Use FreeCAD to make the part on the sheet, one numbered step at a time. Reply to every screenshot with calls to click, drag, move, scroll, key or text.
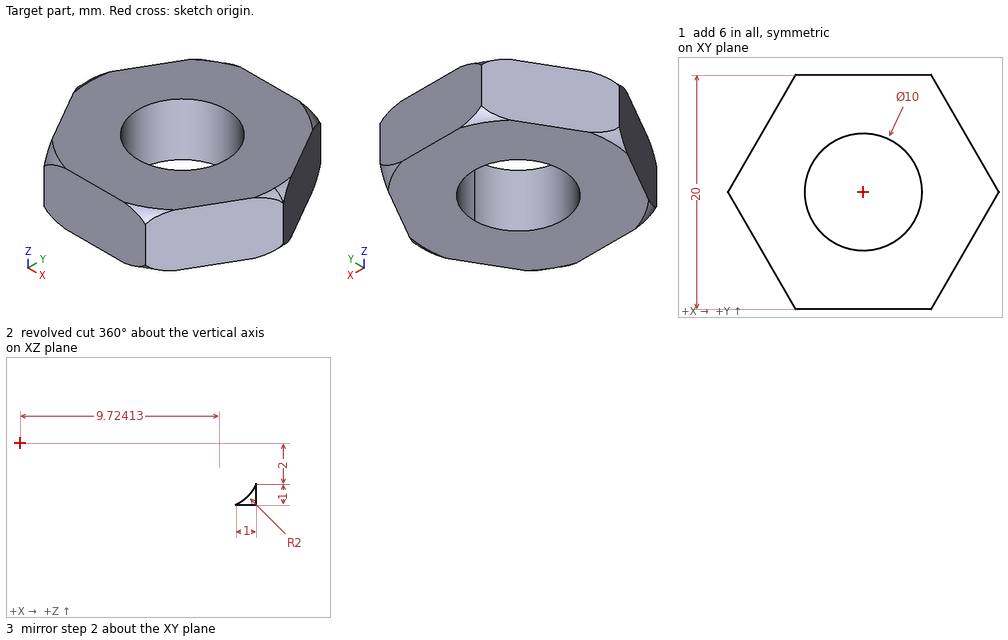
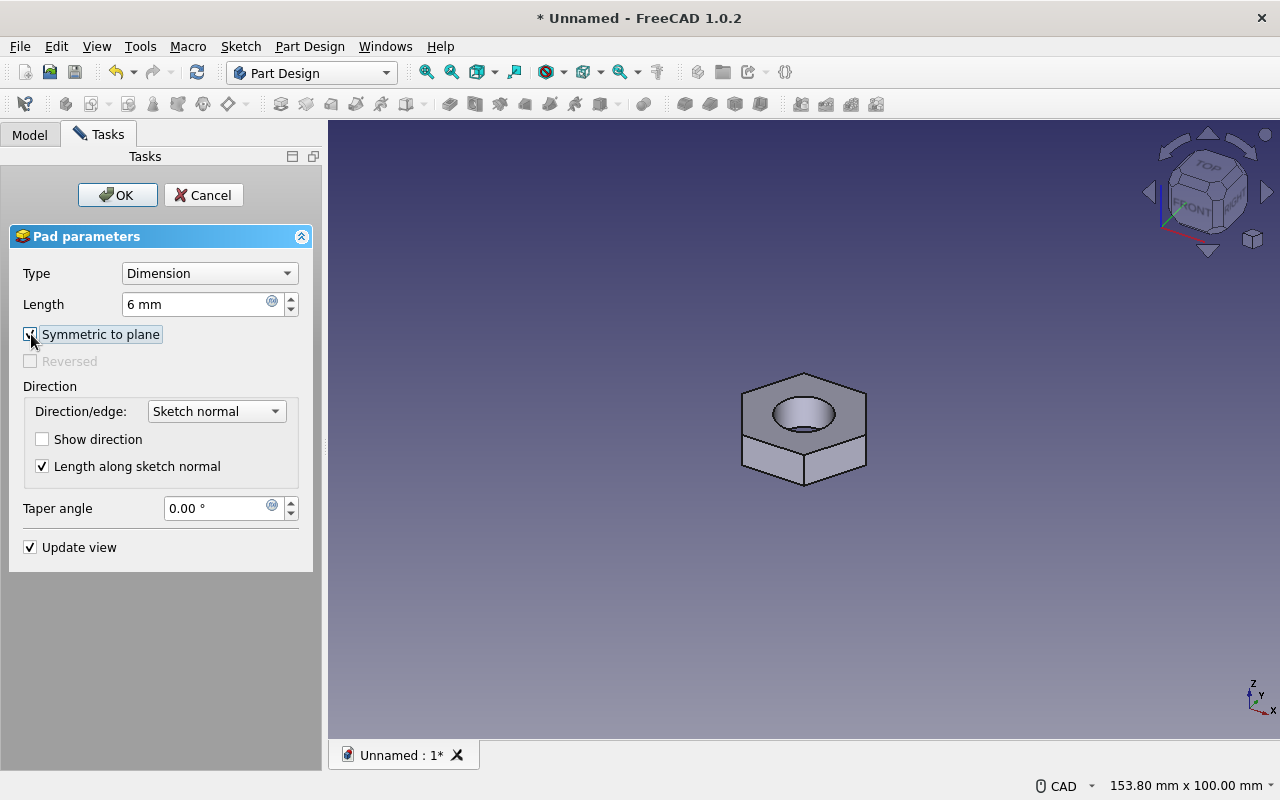
click(118, 195)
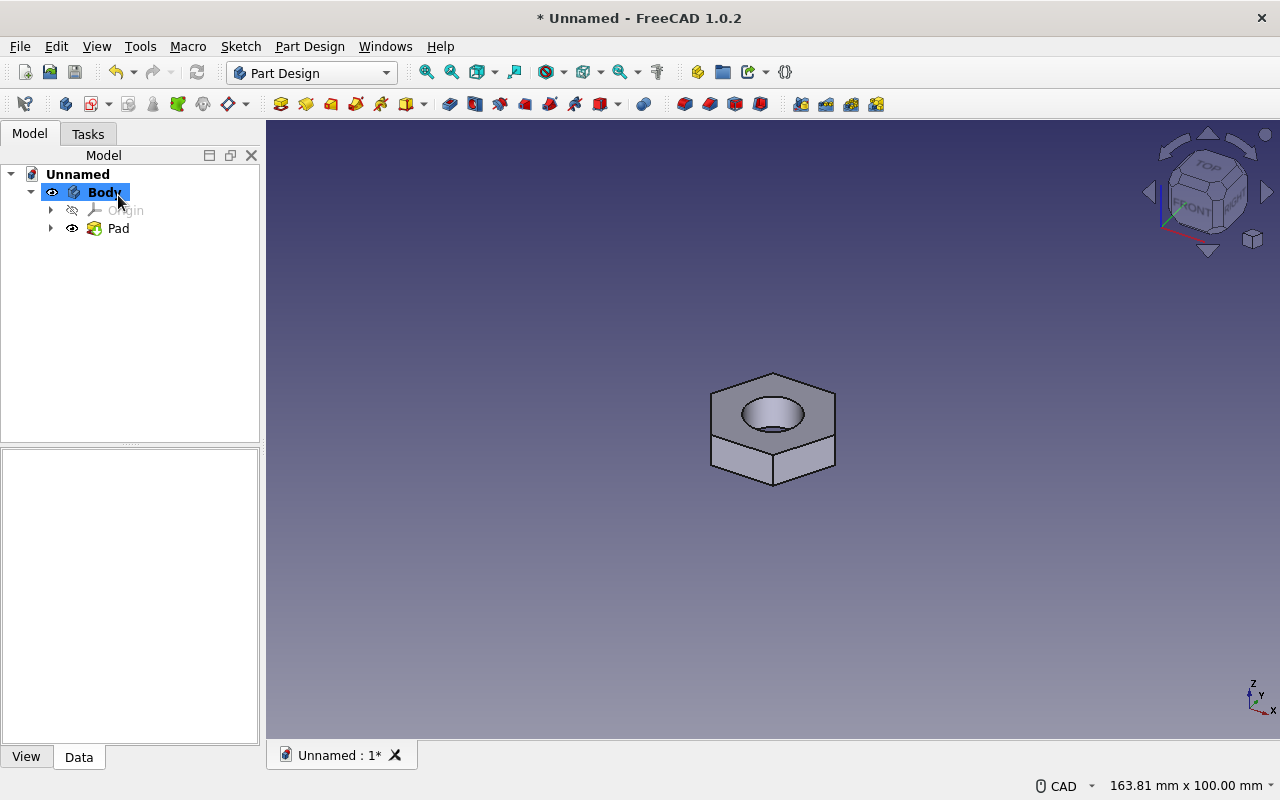
key(v)
key(f)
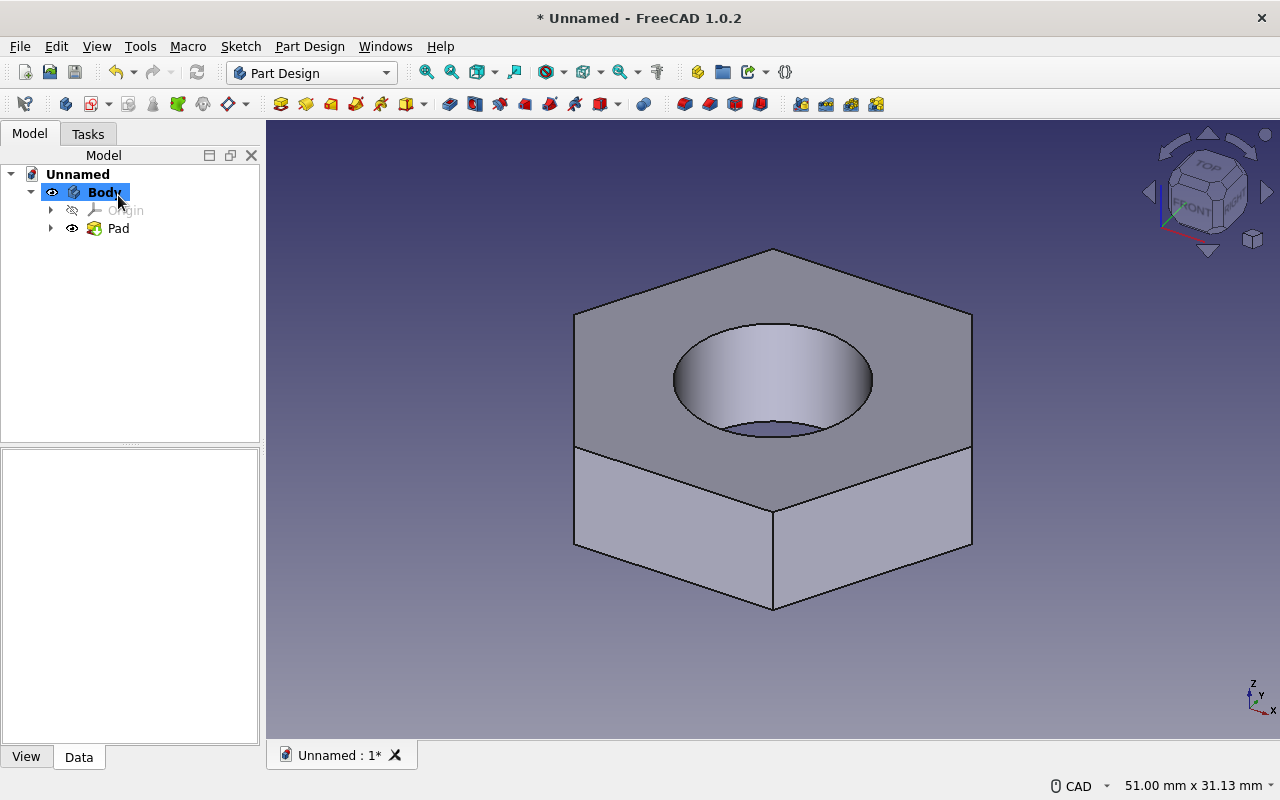
click(90, 104)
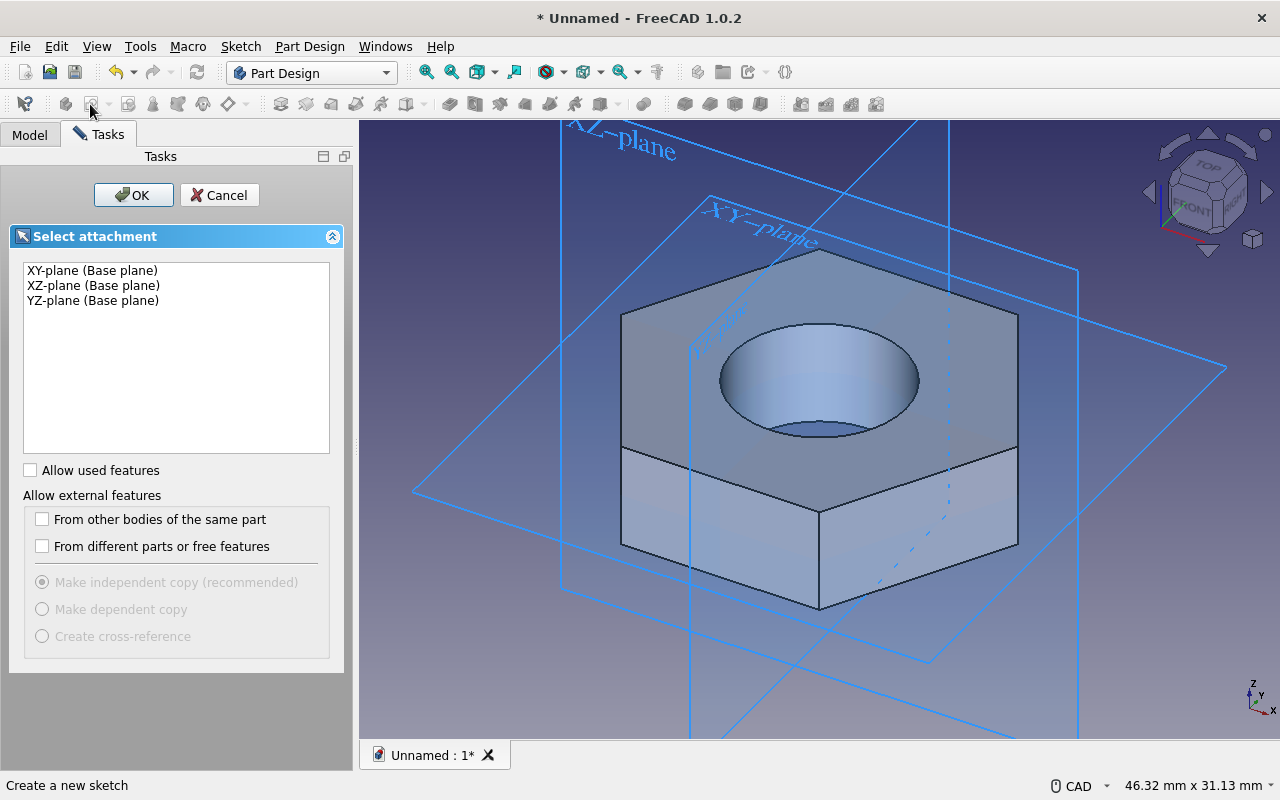
click(84, 286)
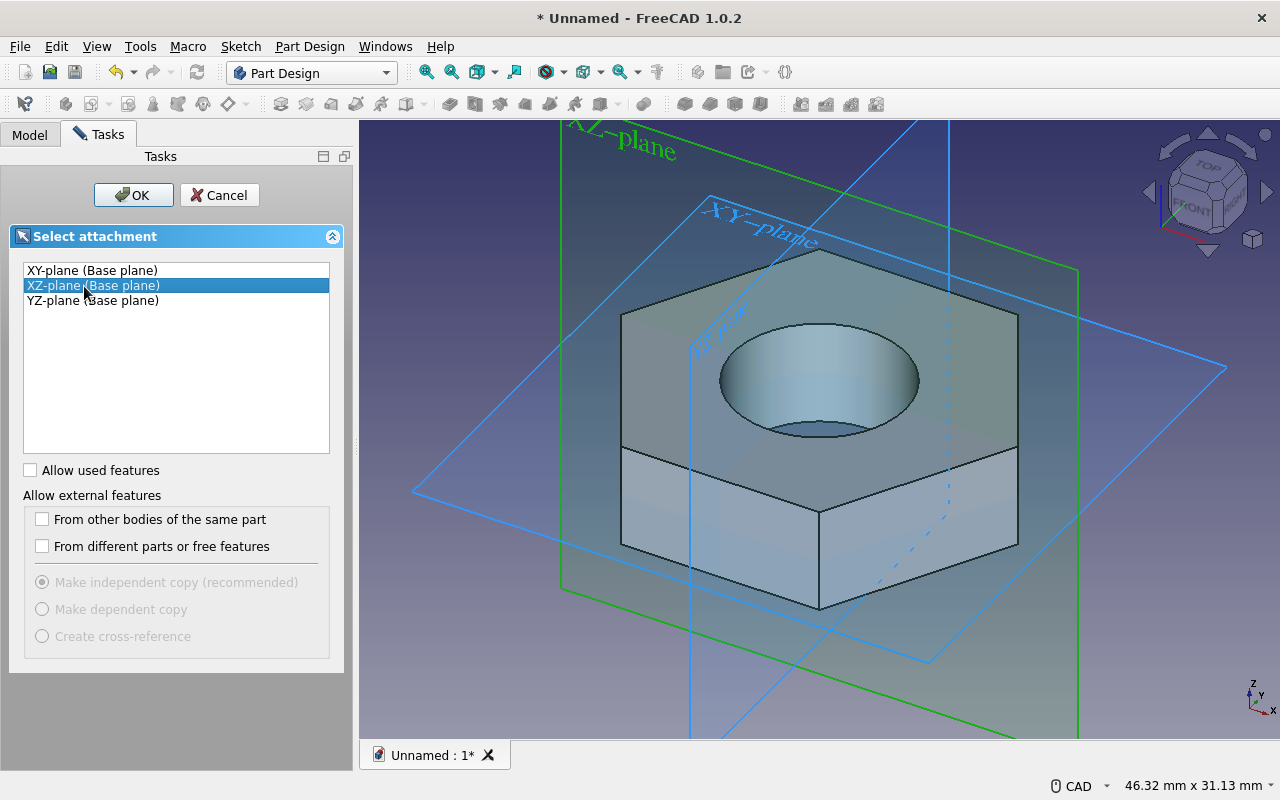
click(134, 195)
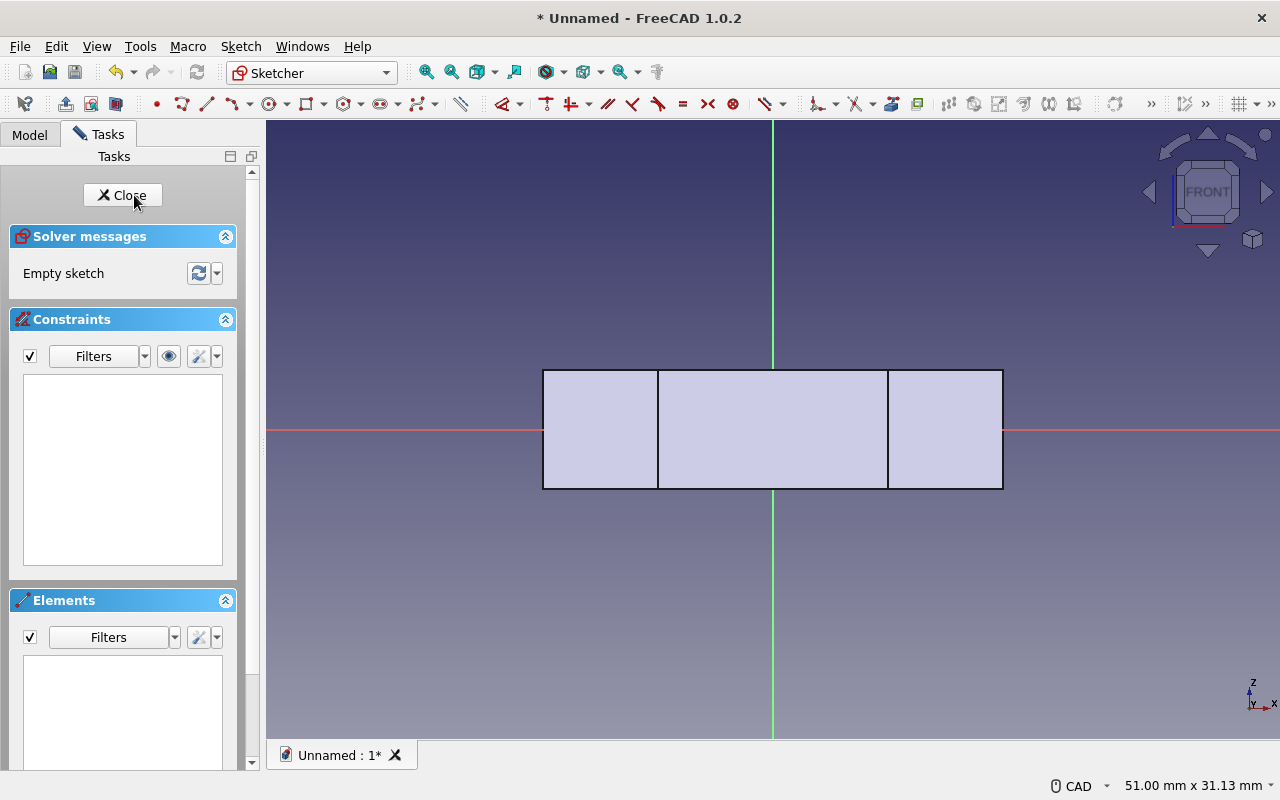
click(116, 104)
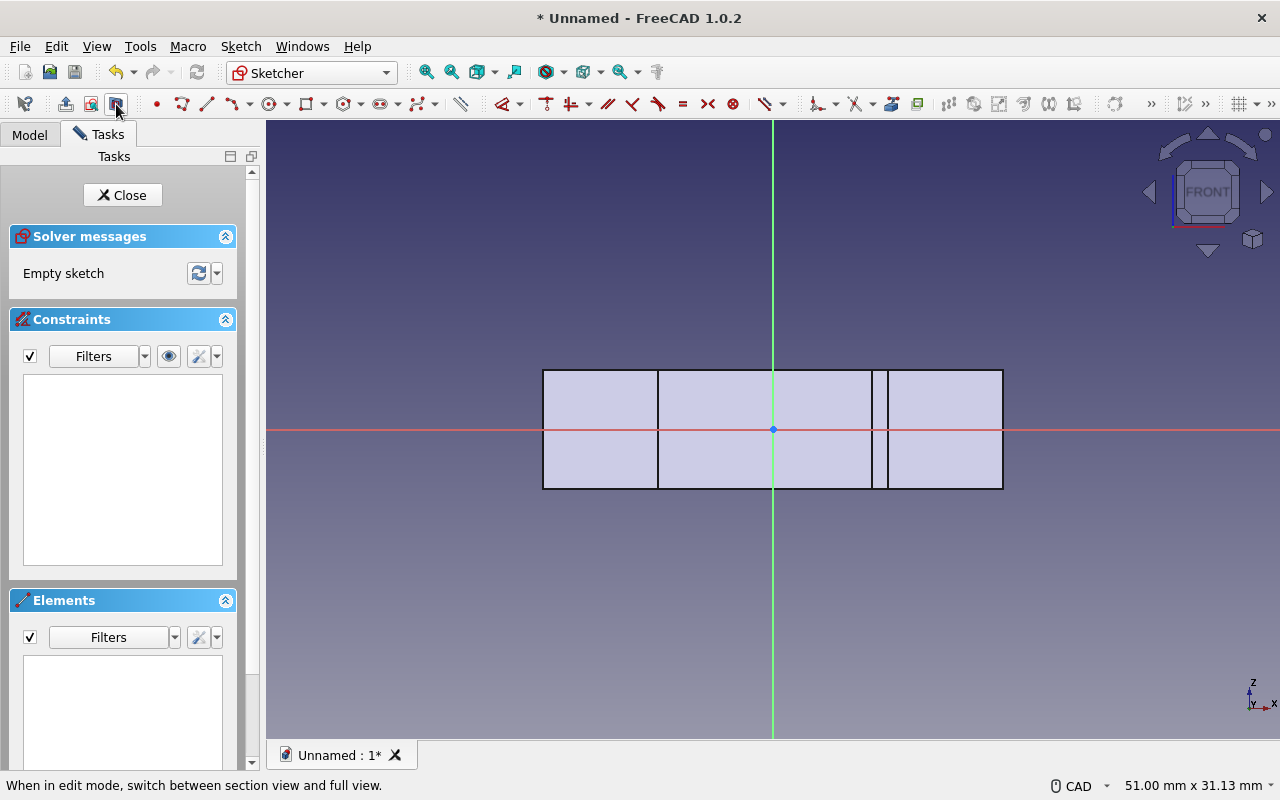
scroll(1008, 482, up, 15)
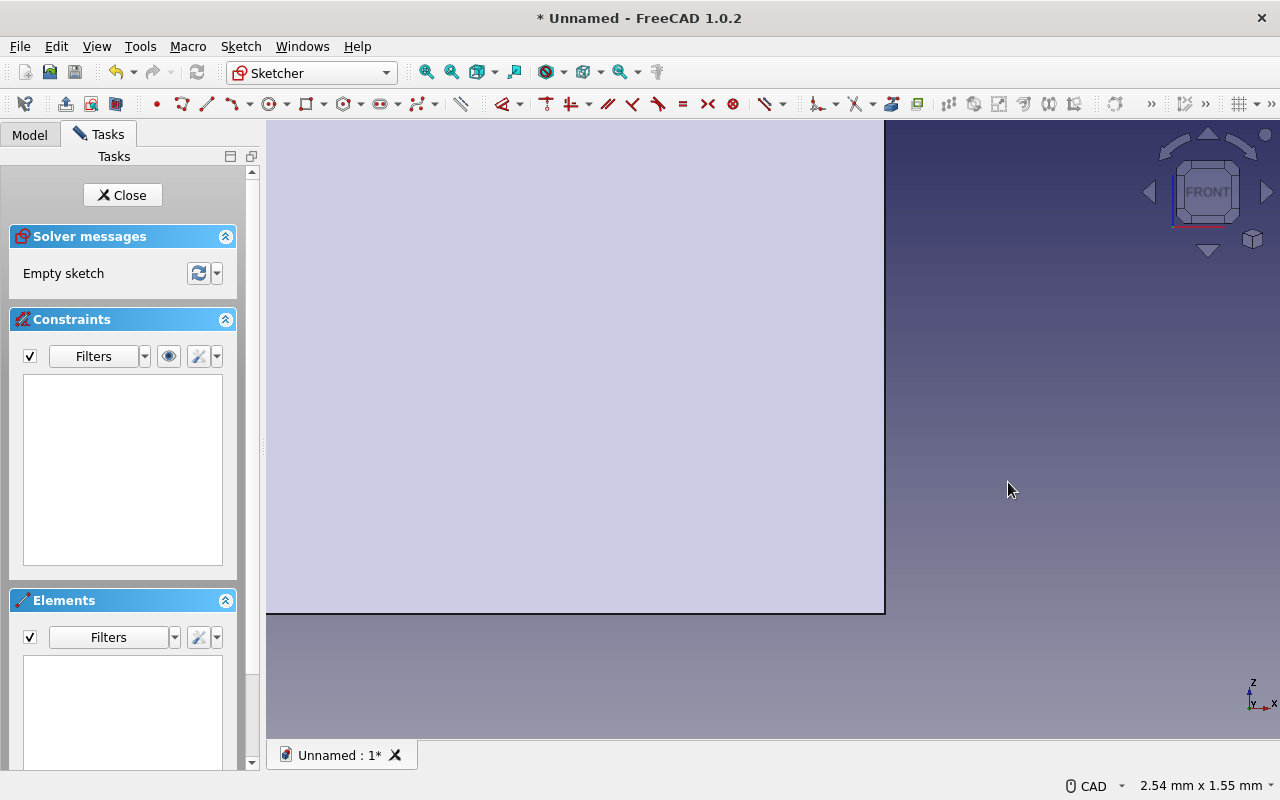
key(g)
key(m)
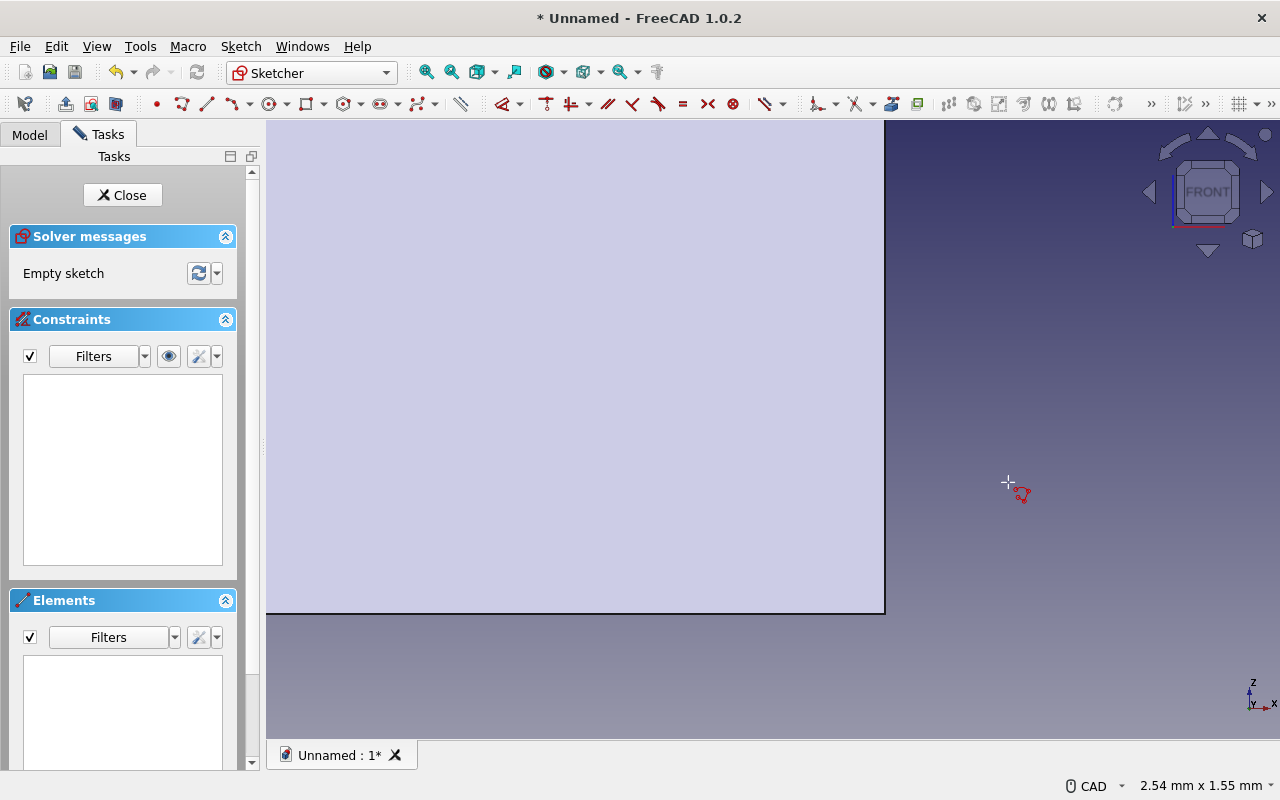
click(885, 215)
click(885, 614)
click(486, 614)
right_click(486, 614)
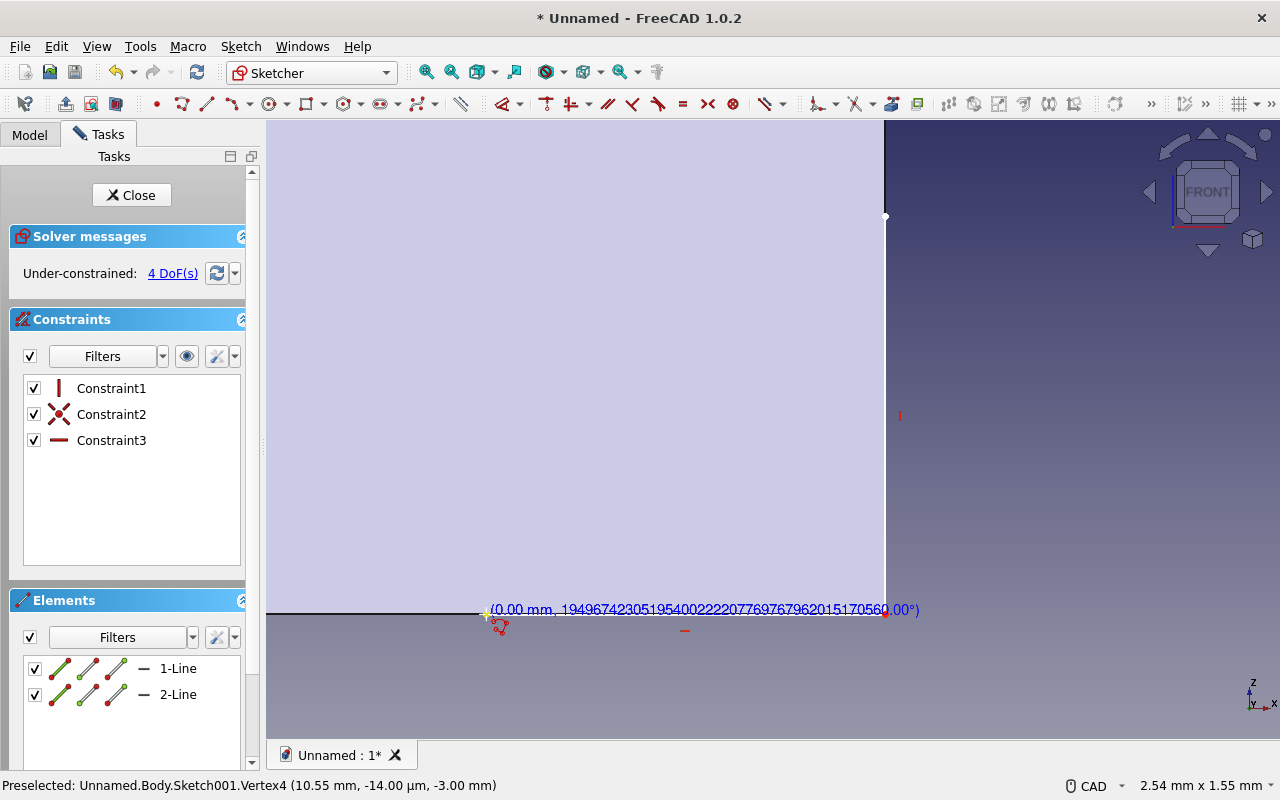
key(g)
key(3)
key(a)